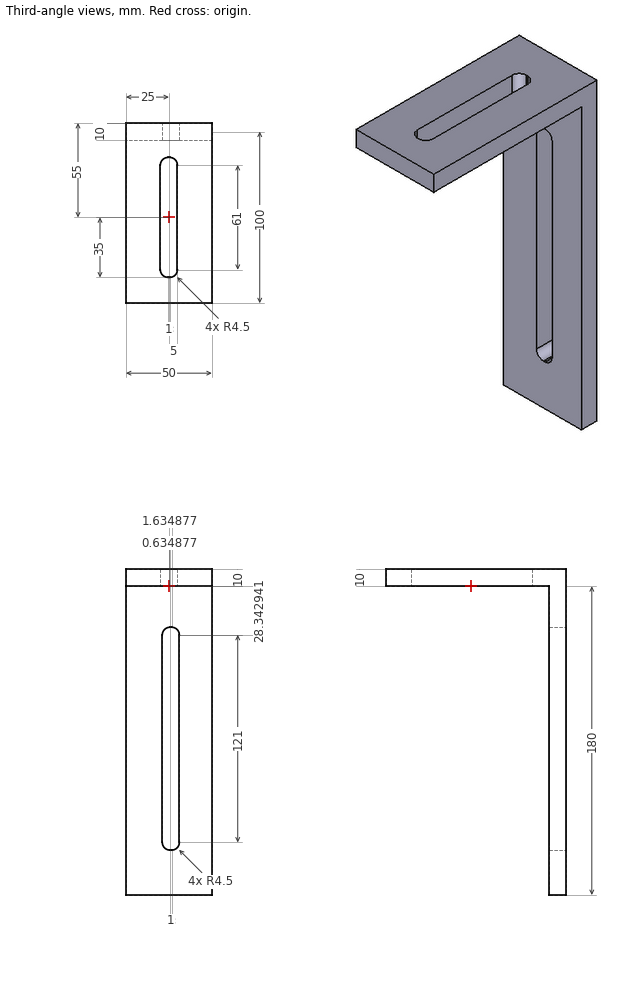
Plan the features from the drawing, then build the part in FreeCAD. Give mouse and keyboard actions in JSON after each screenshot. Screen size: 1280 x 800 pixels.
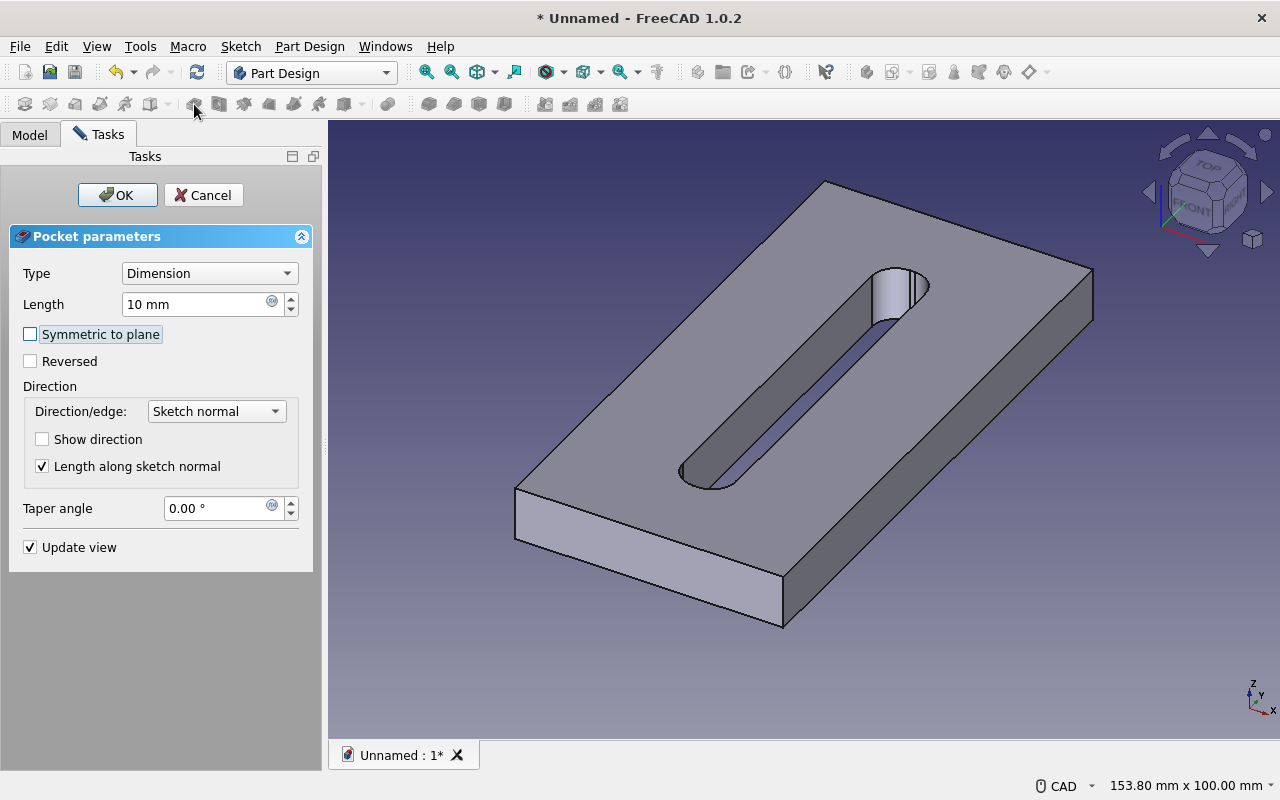
{"action": "left_click", "coordinate": [118, 195]}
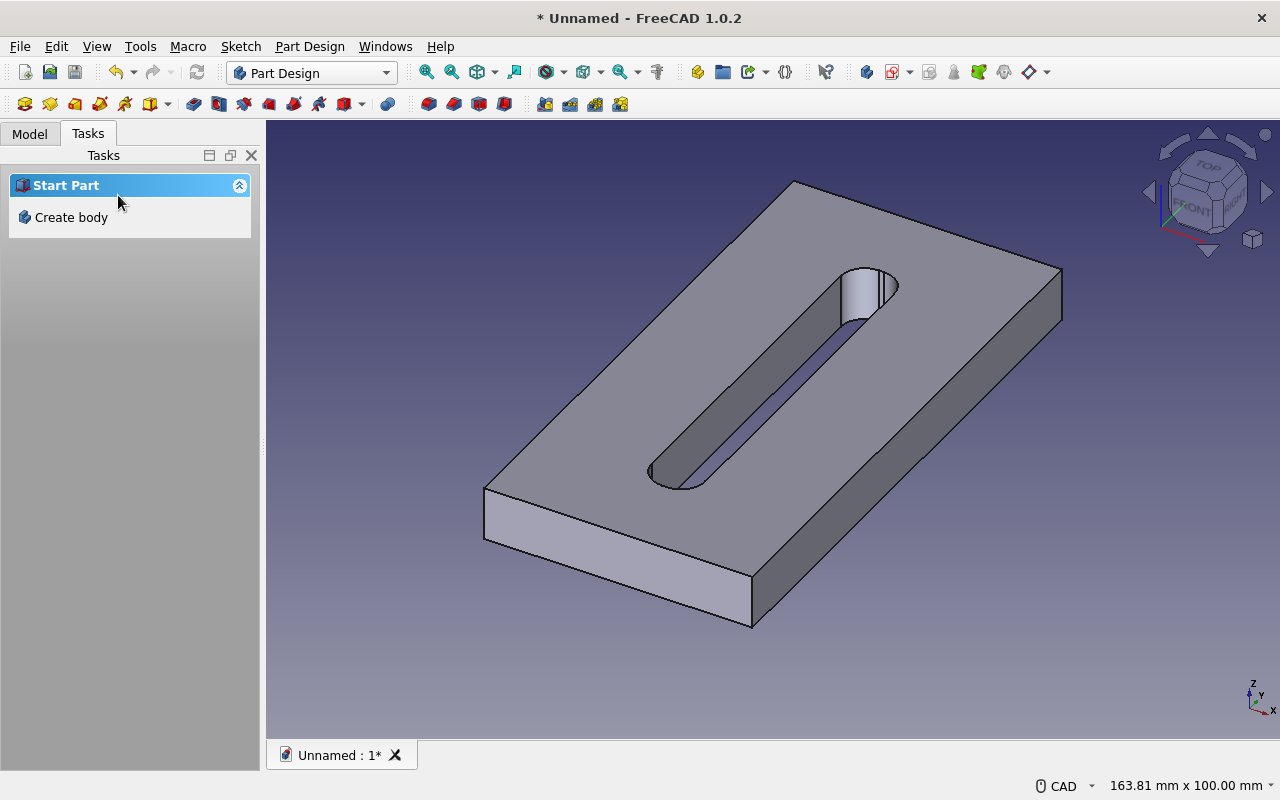
{"action": "left_click", "coordinate": [892, 72]}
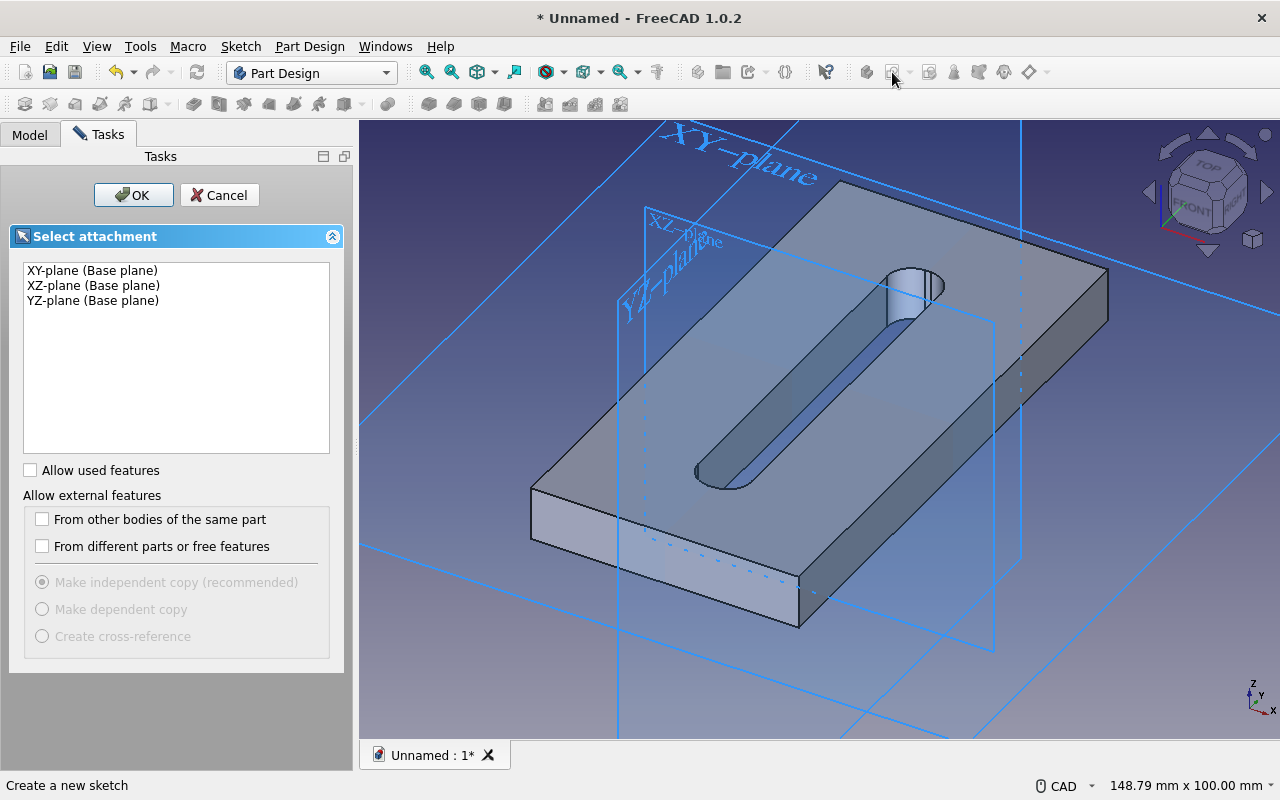
{"action": "left_click", "coordinate": [84, 270]}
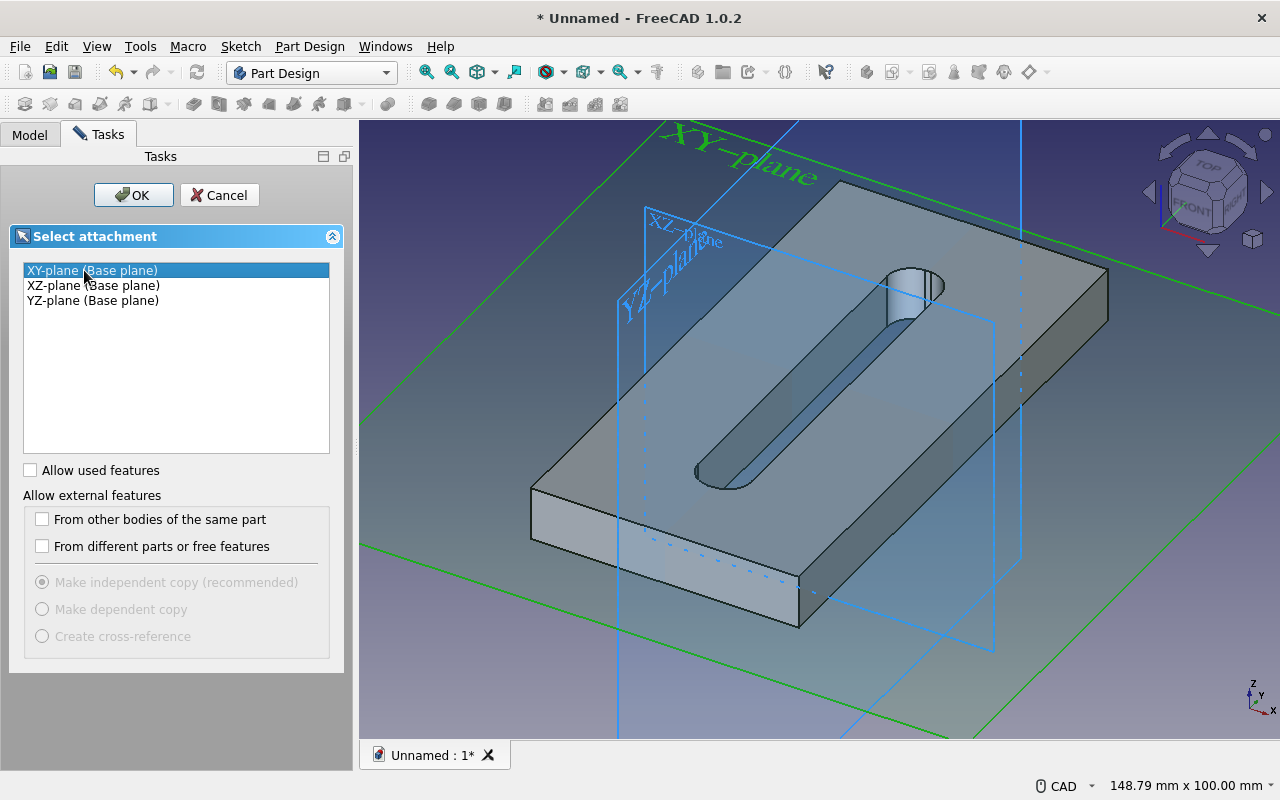
{"action": "left_click", "coordinate": [134, 195]}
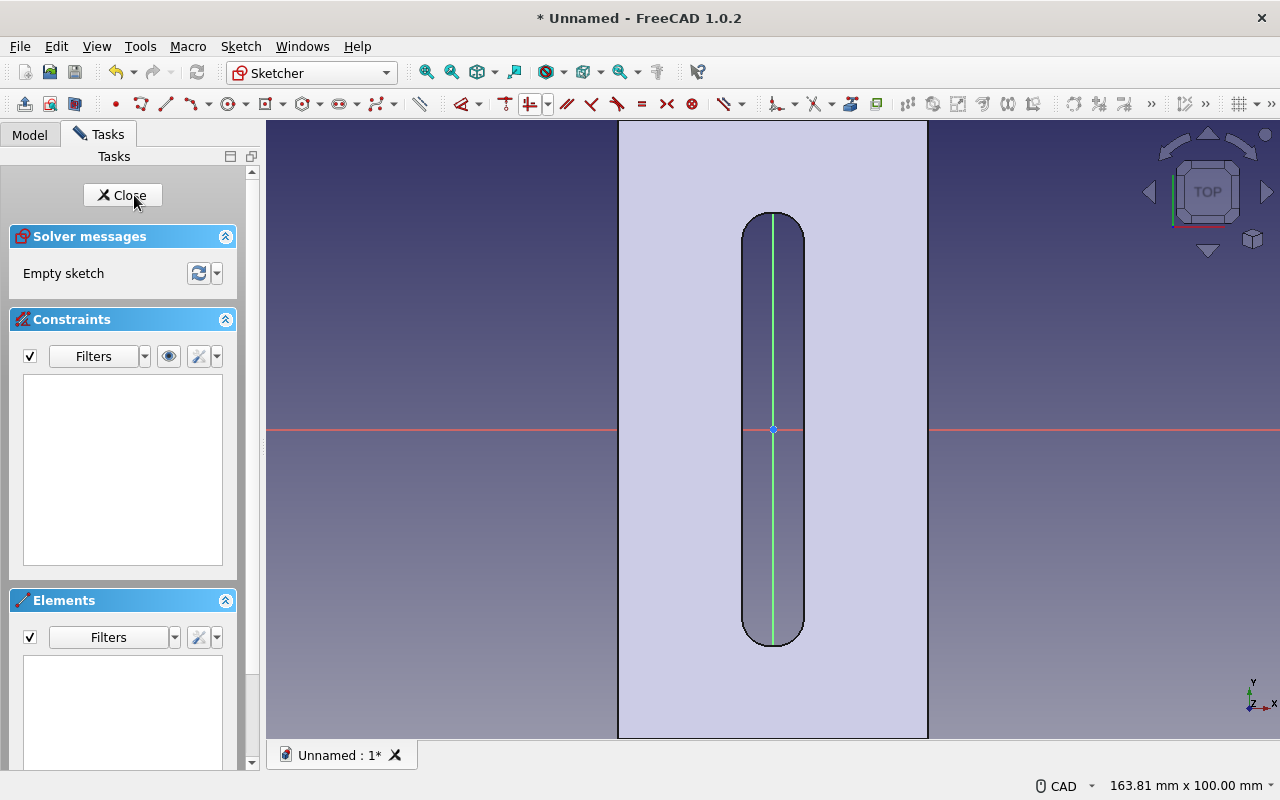
{"action": "left_click", "coordinate": [75, 104]}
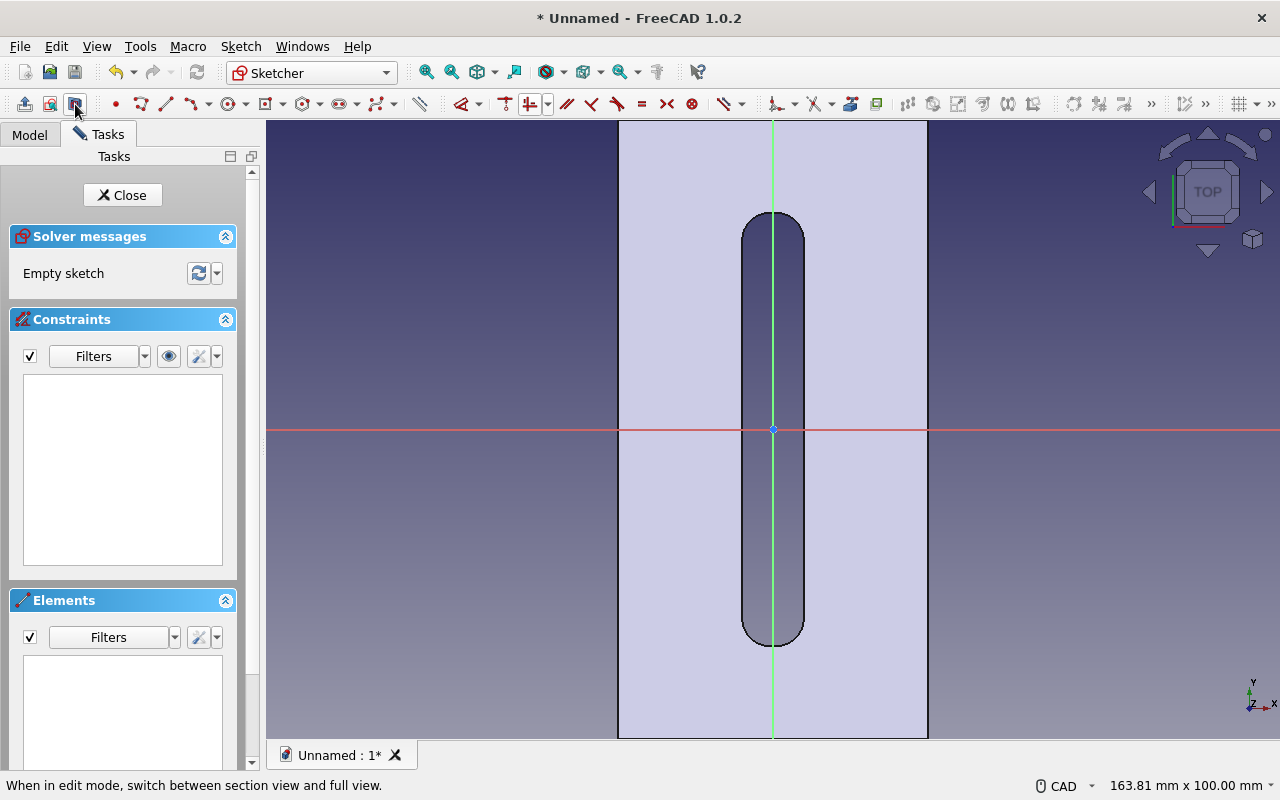
{"action": "scroll", "coordinate": [395, 711], "scroll_direction": "down", "scroll_amount": 1}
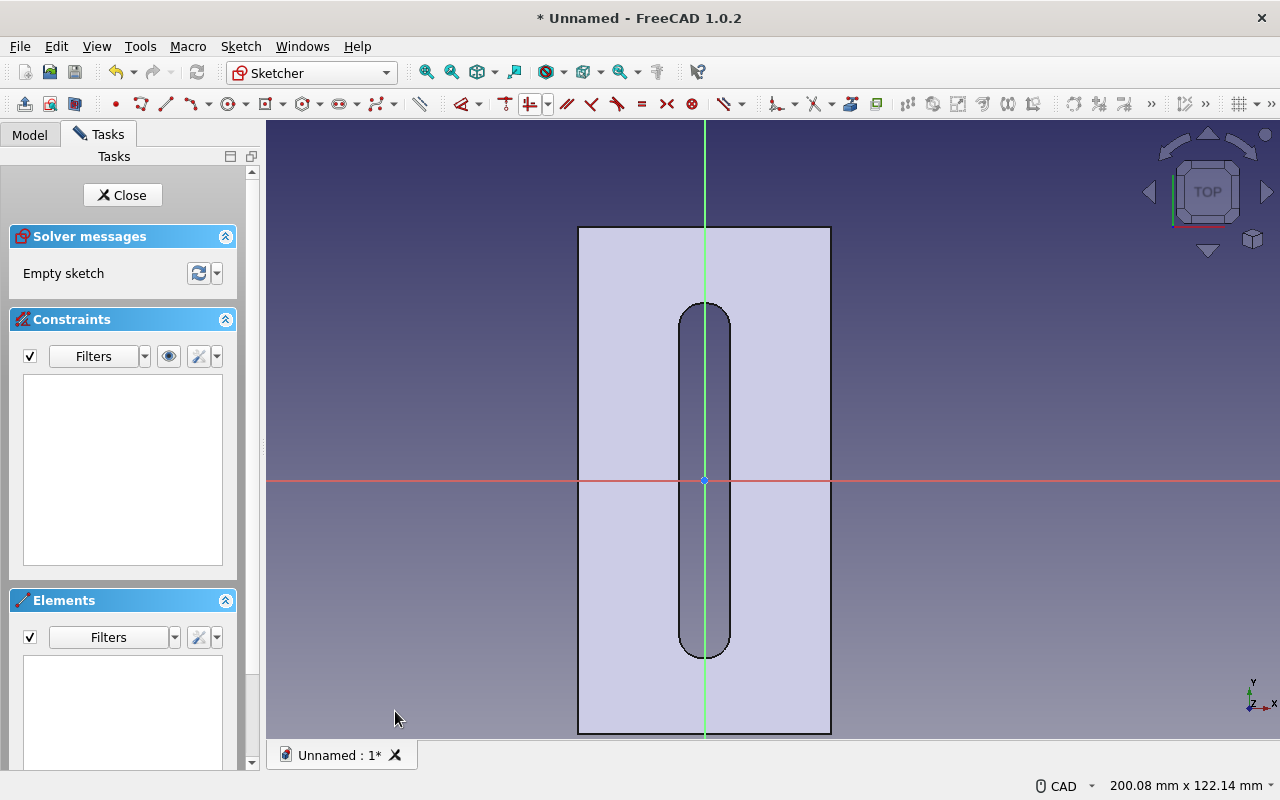
{"action": "scroll", "coordinate": [705, 162], "scroll_direction": "up", "scroll_amount": 2}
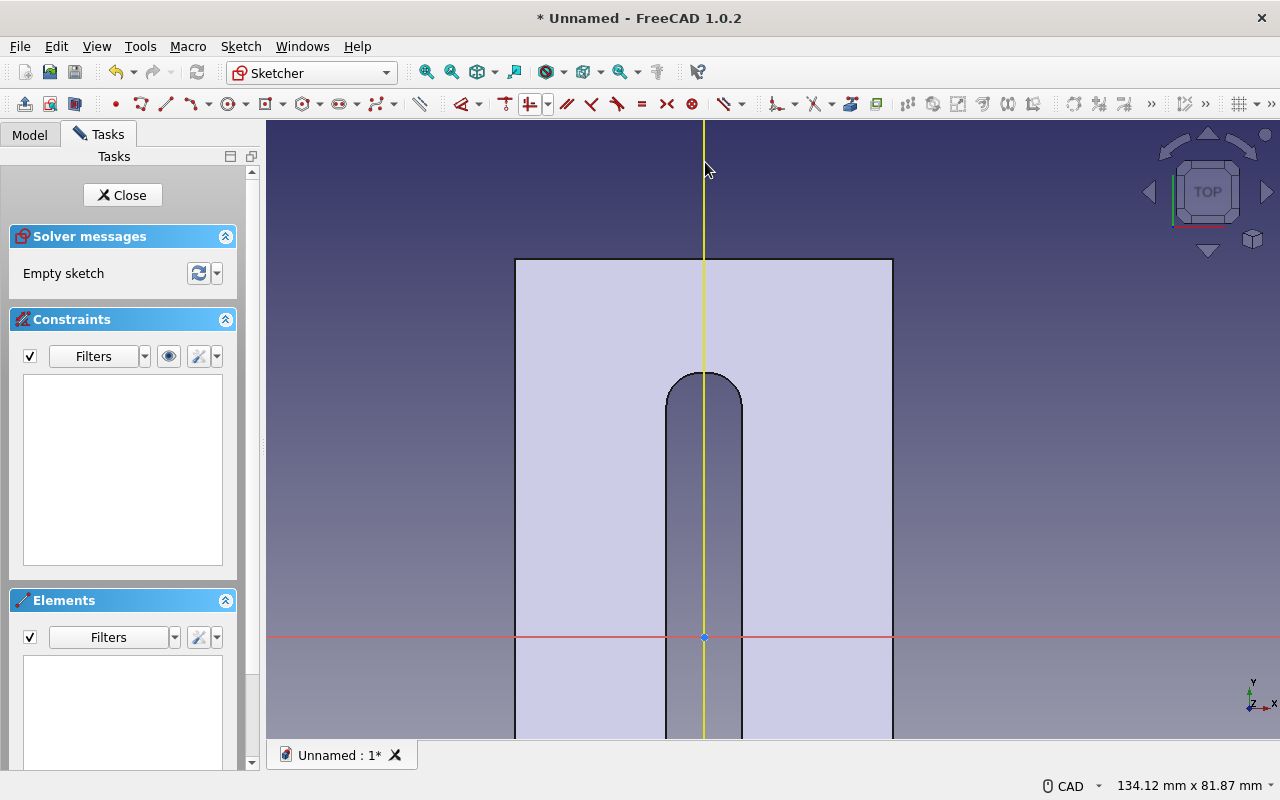
{"action": "left_click", "coordinate": [282, 104]}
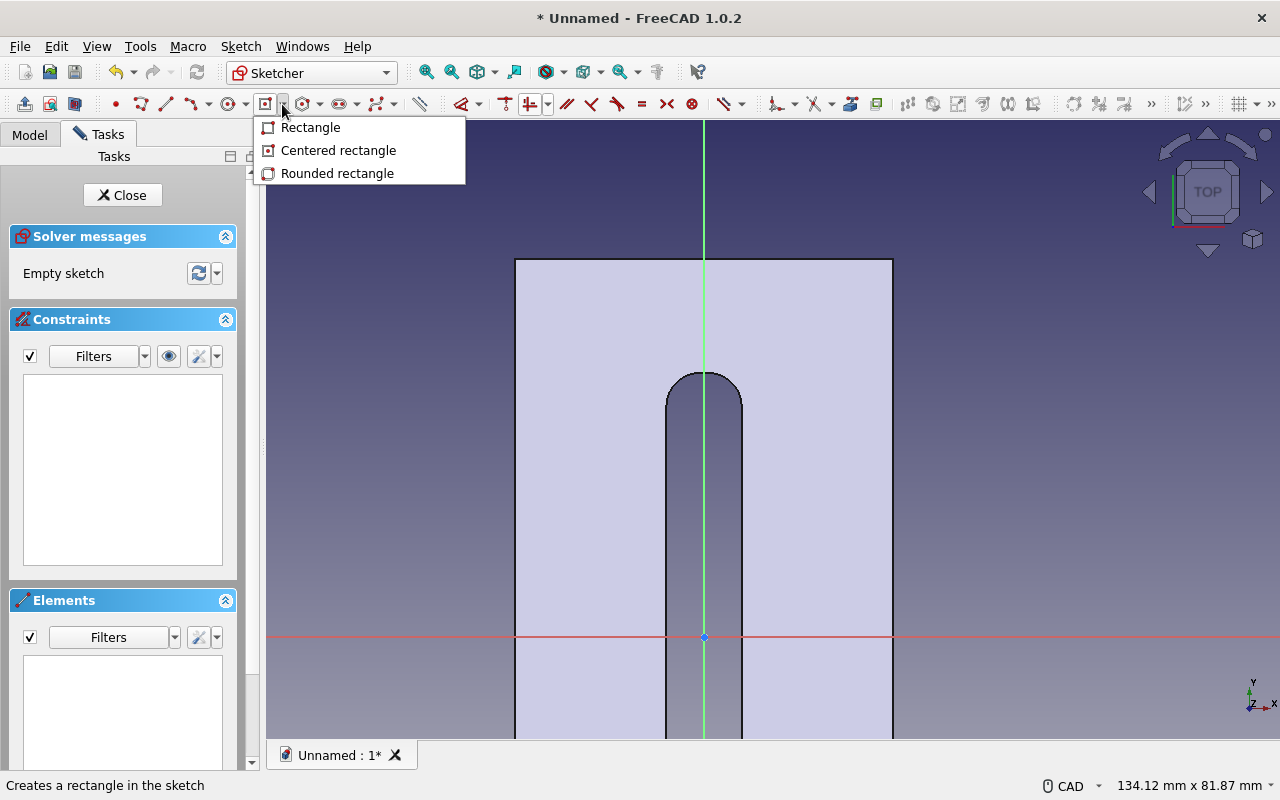
{"action": "left_click", "coordinate": [360, 128]}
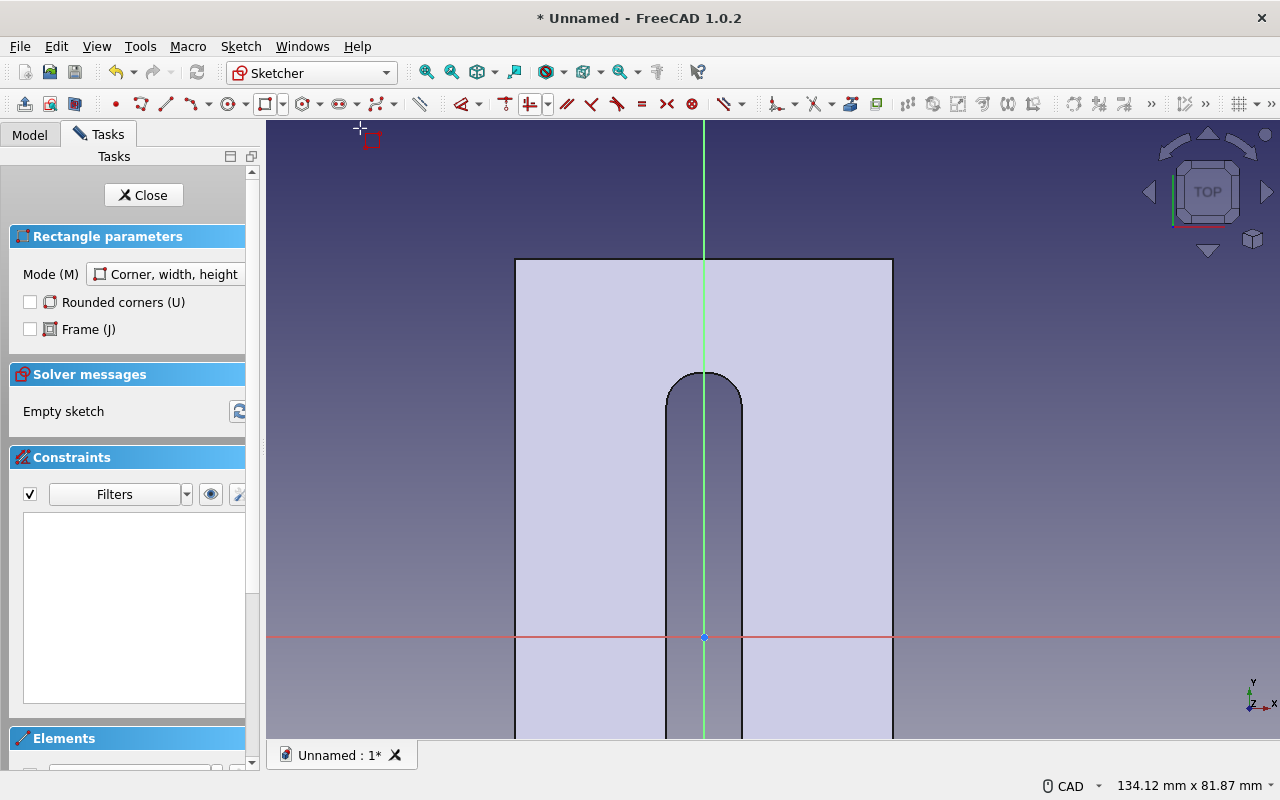
{"action": "left_click", "coordinate": [515, 222]}
{"action": "left_click", "coordinate": [893, 297]}
{"action": "key", "text": "Escape"}